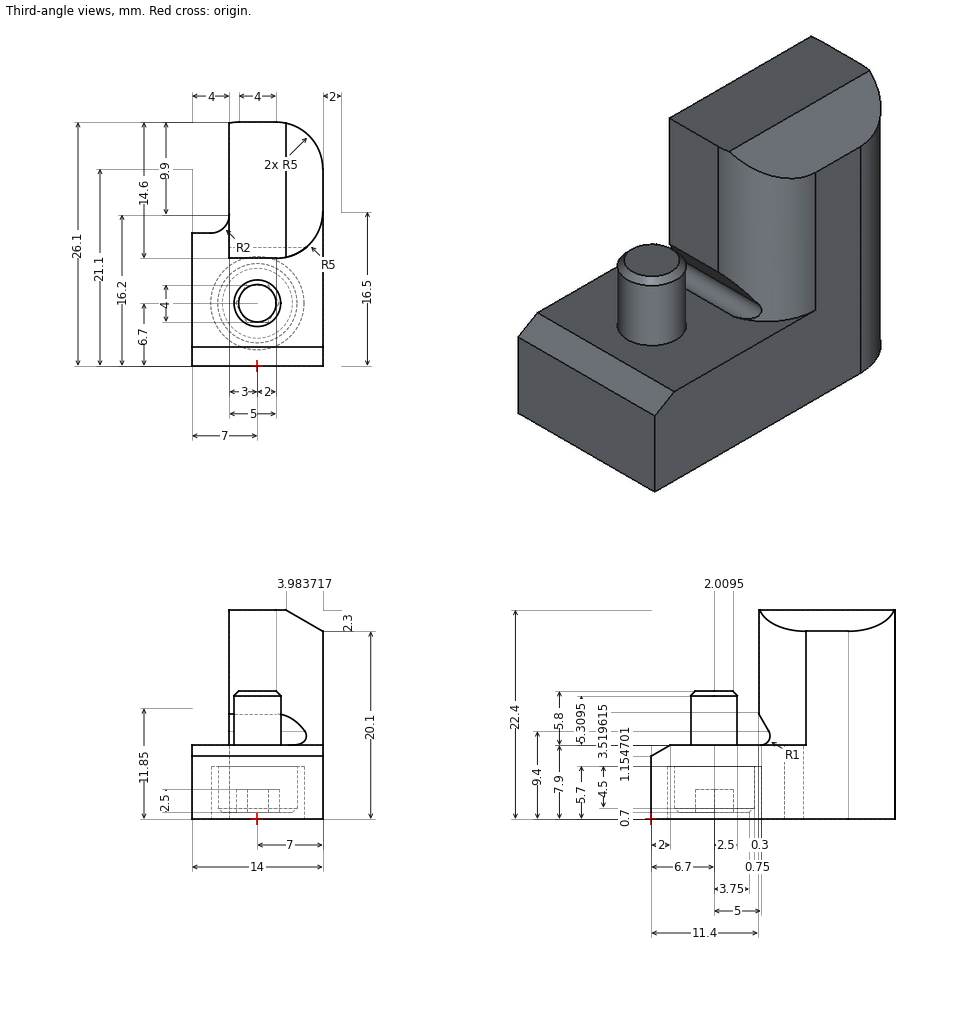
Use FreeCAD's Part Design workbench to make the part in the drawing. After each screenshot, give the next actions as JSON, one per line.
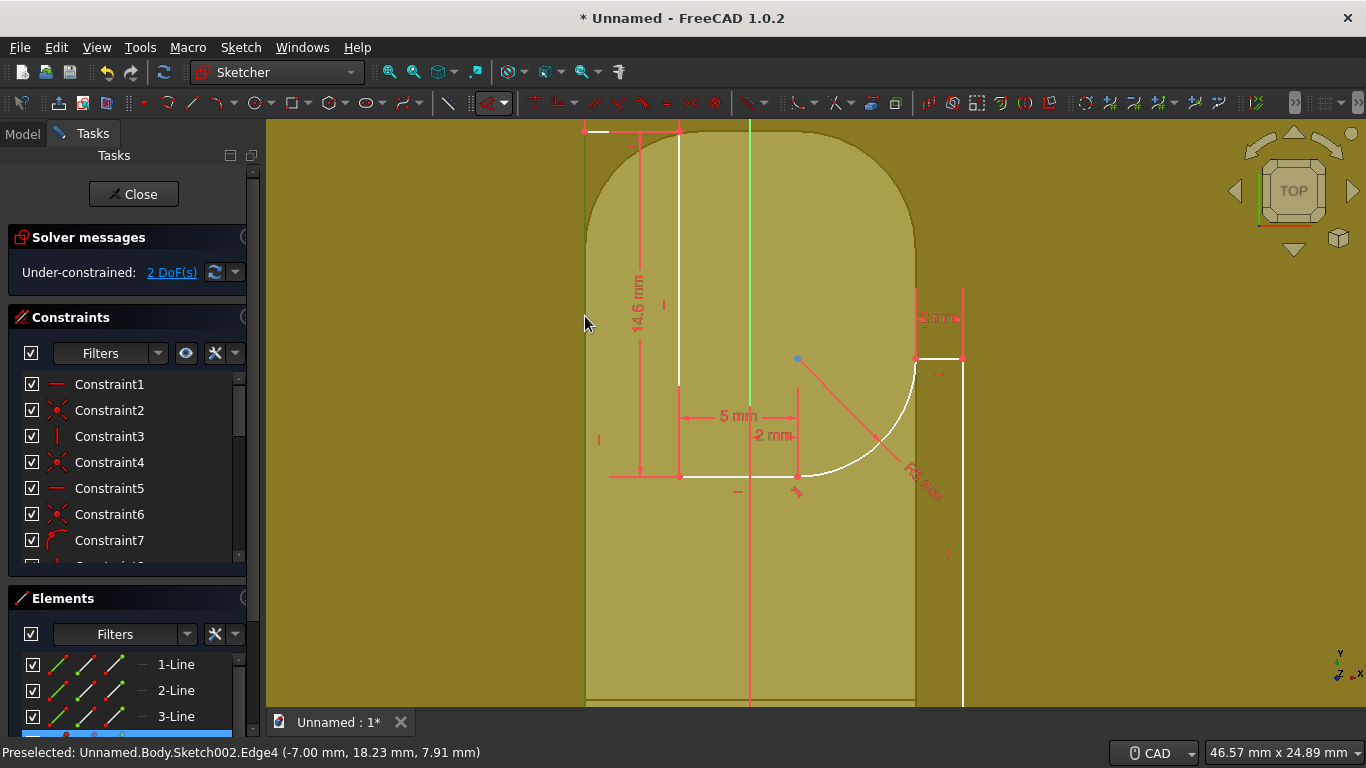
{"action": "left_click", "coordinate": [506, 104]}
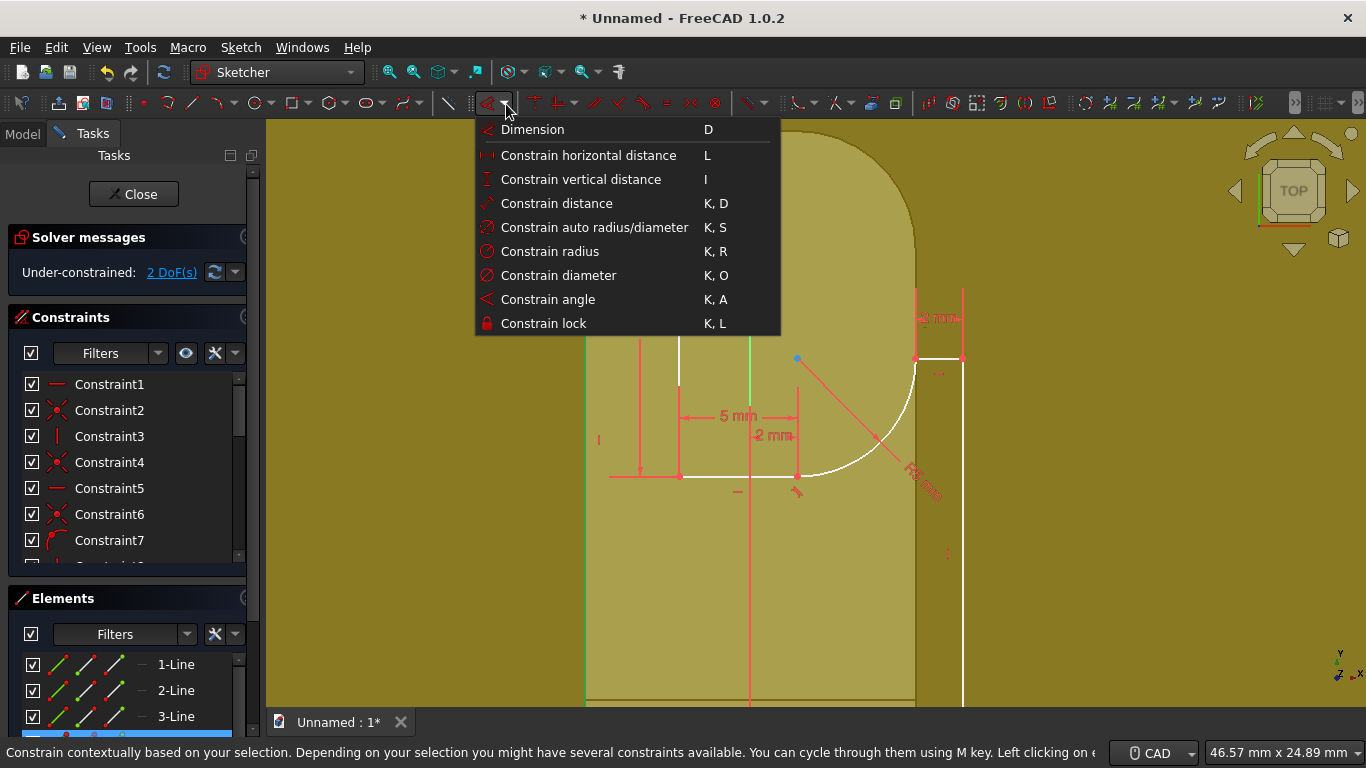
{"action": "left_click", "coordinate": [628, 179]}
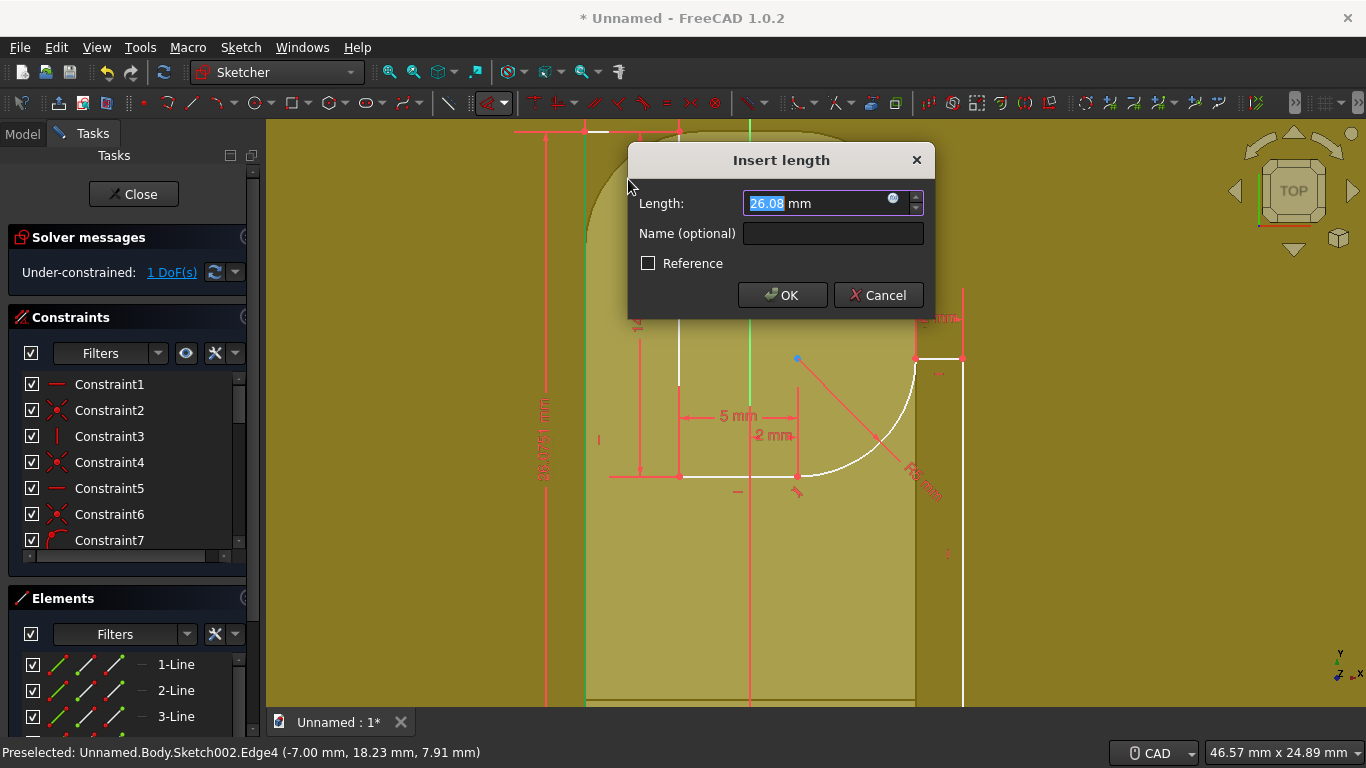
{"action": "type", "text": "26.1"}
{"action": "key", "text": "Return"}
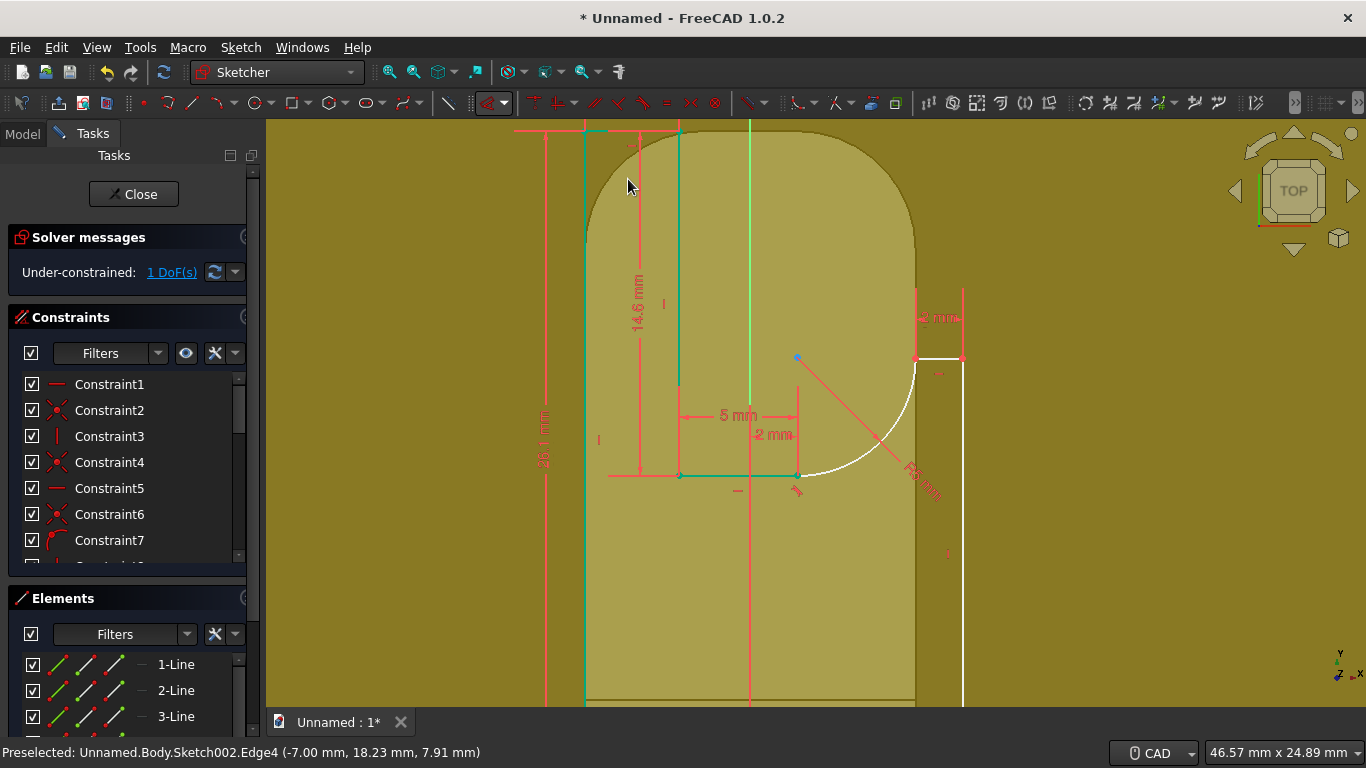
{"action": "left_click", "coordinate": [963, 631]}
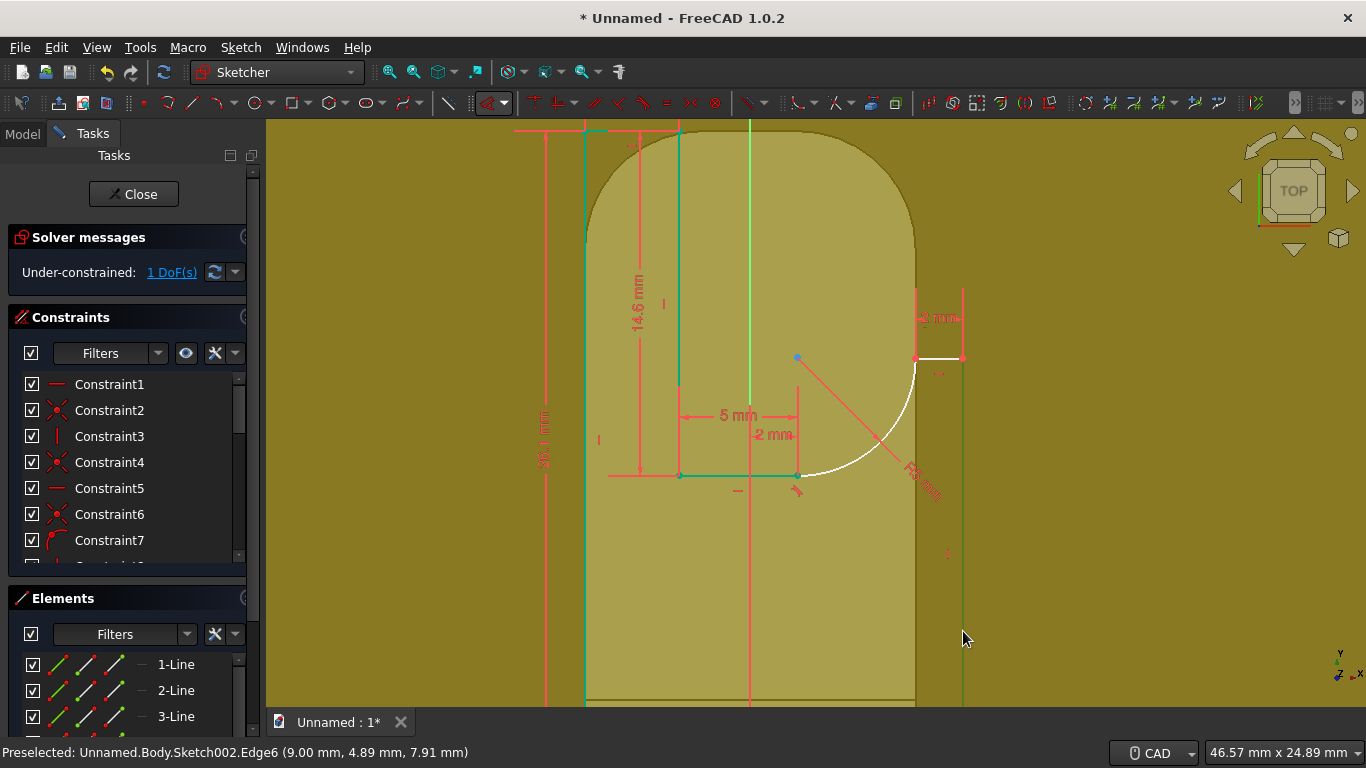
{"action": "left_click", "coordinate": [506, 104]}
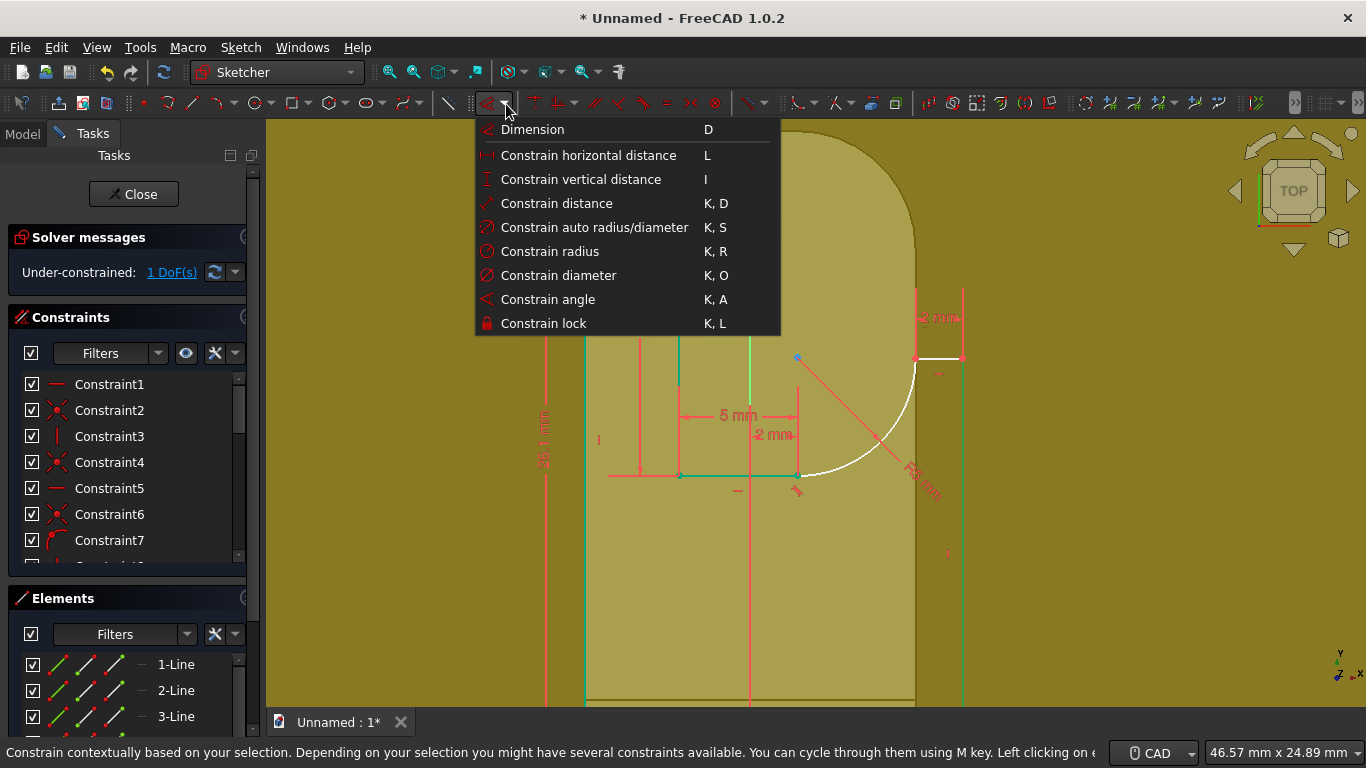
{"action": "left_click", "coordinate": [628, 179]}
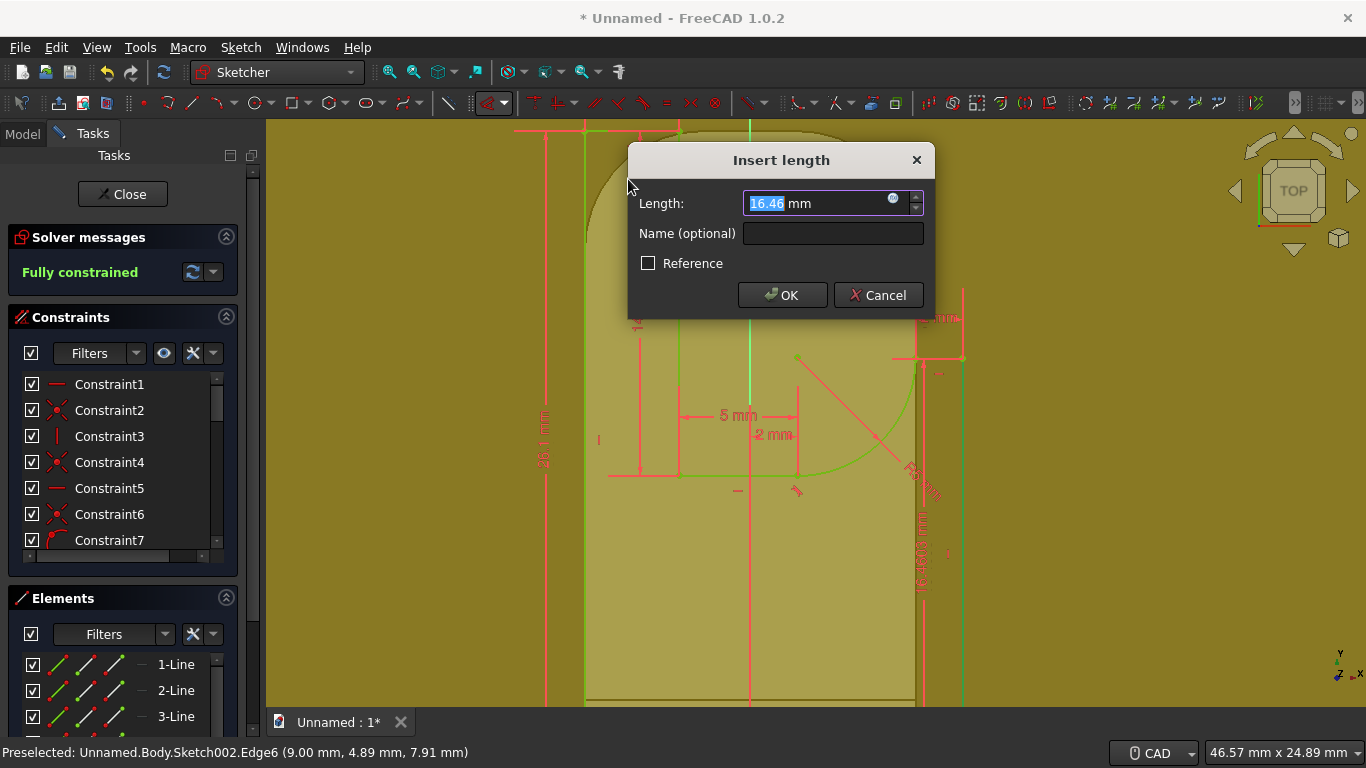
{"action": "type", "text": "16.5"}
{"action": "key", "text": "Return"}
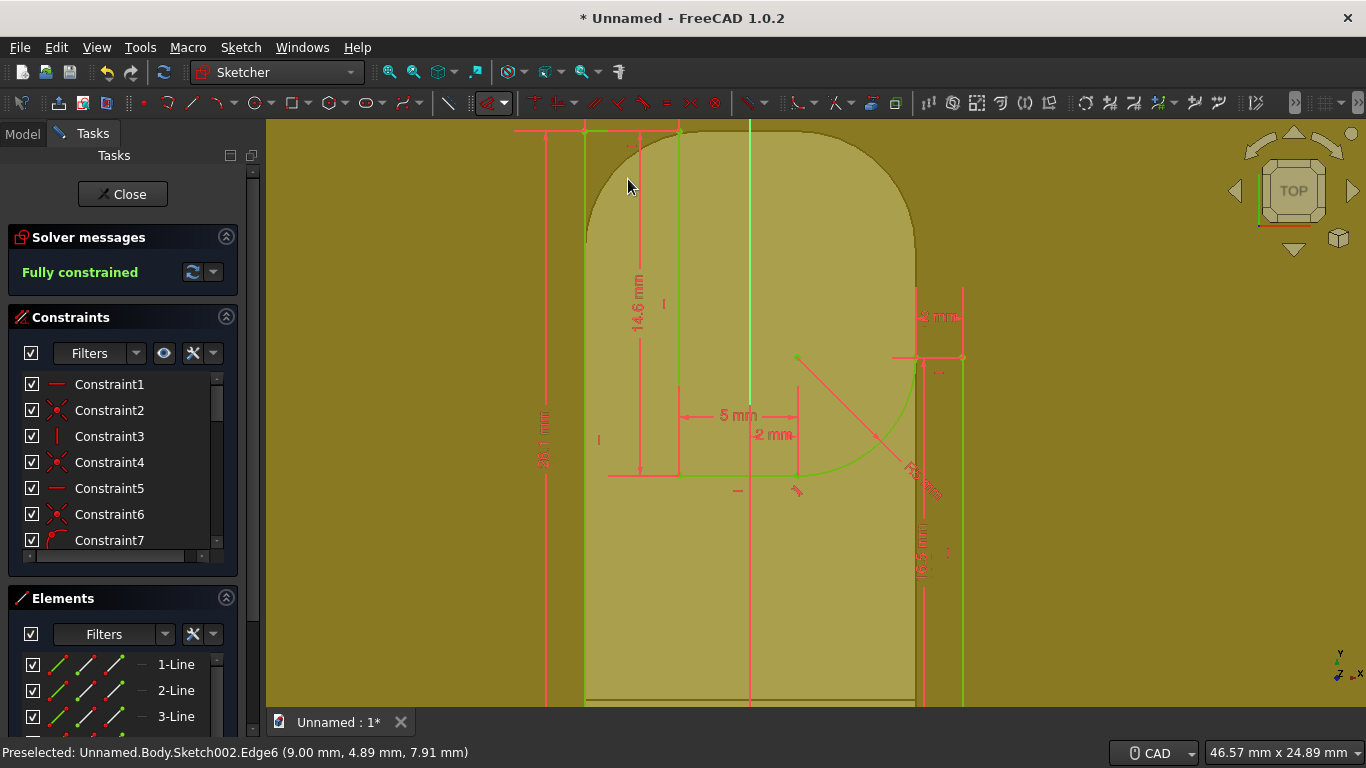
{"action": "left_click", "coordinate": [123, 194]}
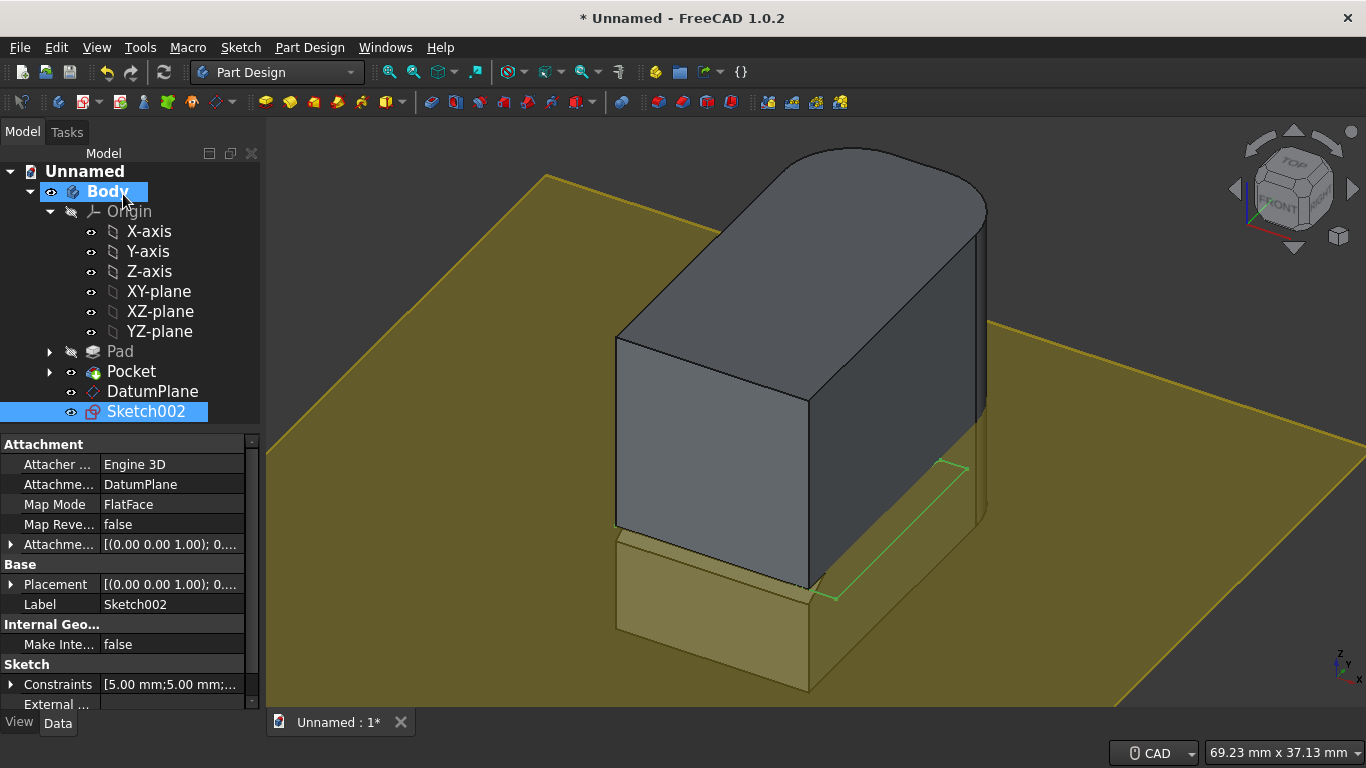
{"action": "left_click", "coordinate": [432, 102]}